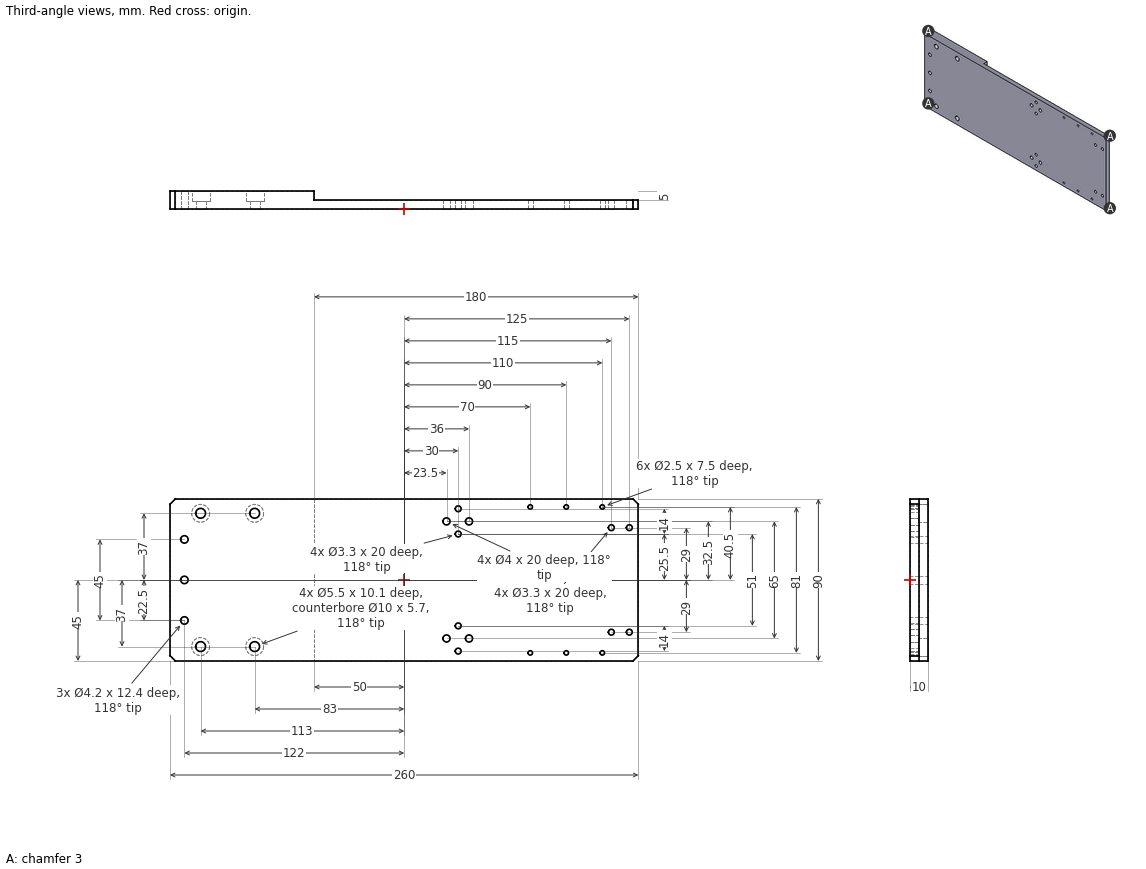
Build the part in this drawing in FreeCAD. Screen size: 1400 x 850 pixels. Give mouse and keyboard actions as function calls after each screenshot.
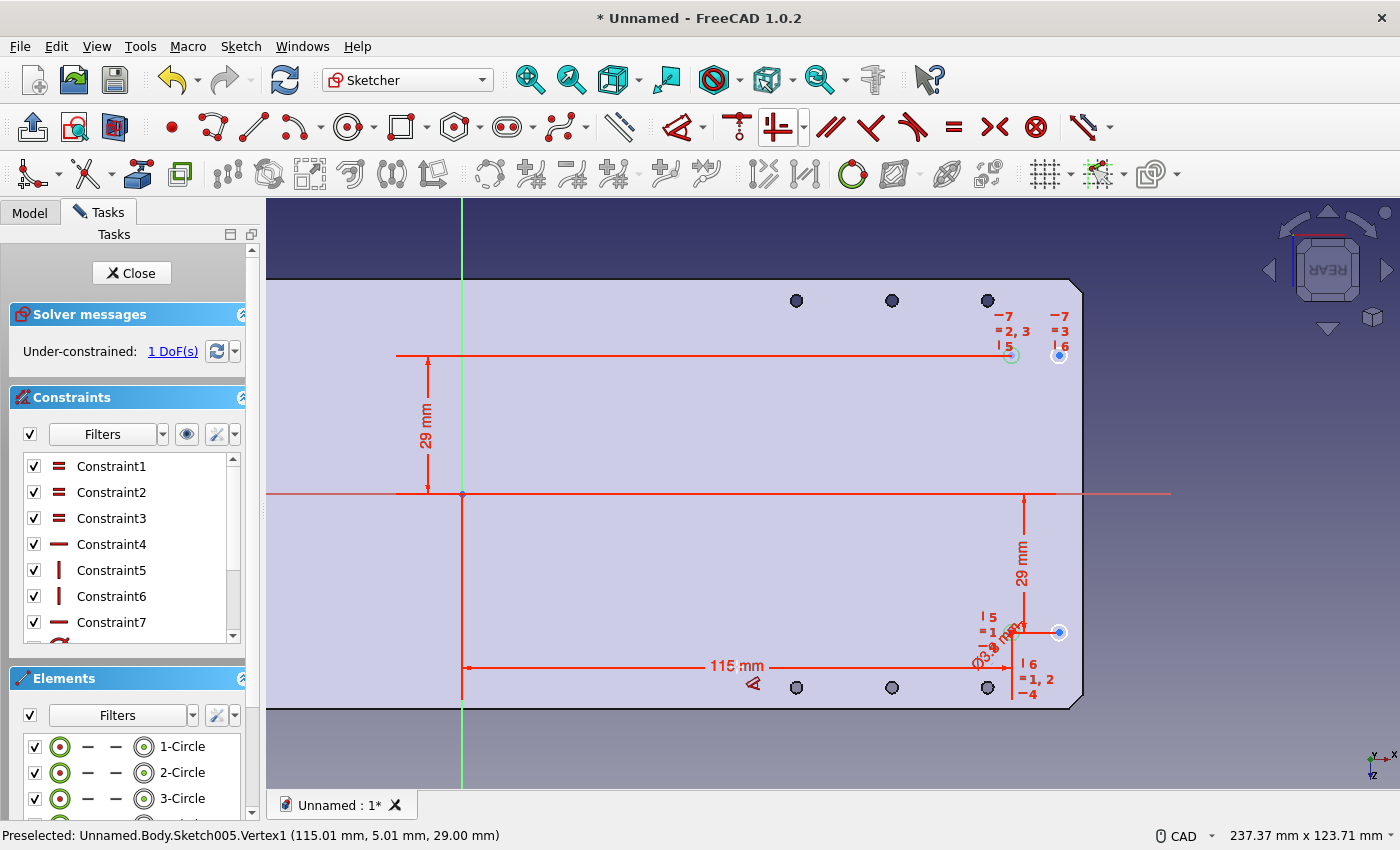
click(1059, 633)
click(623, 667)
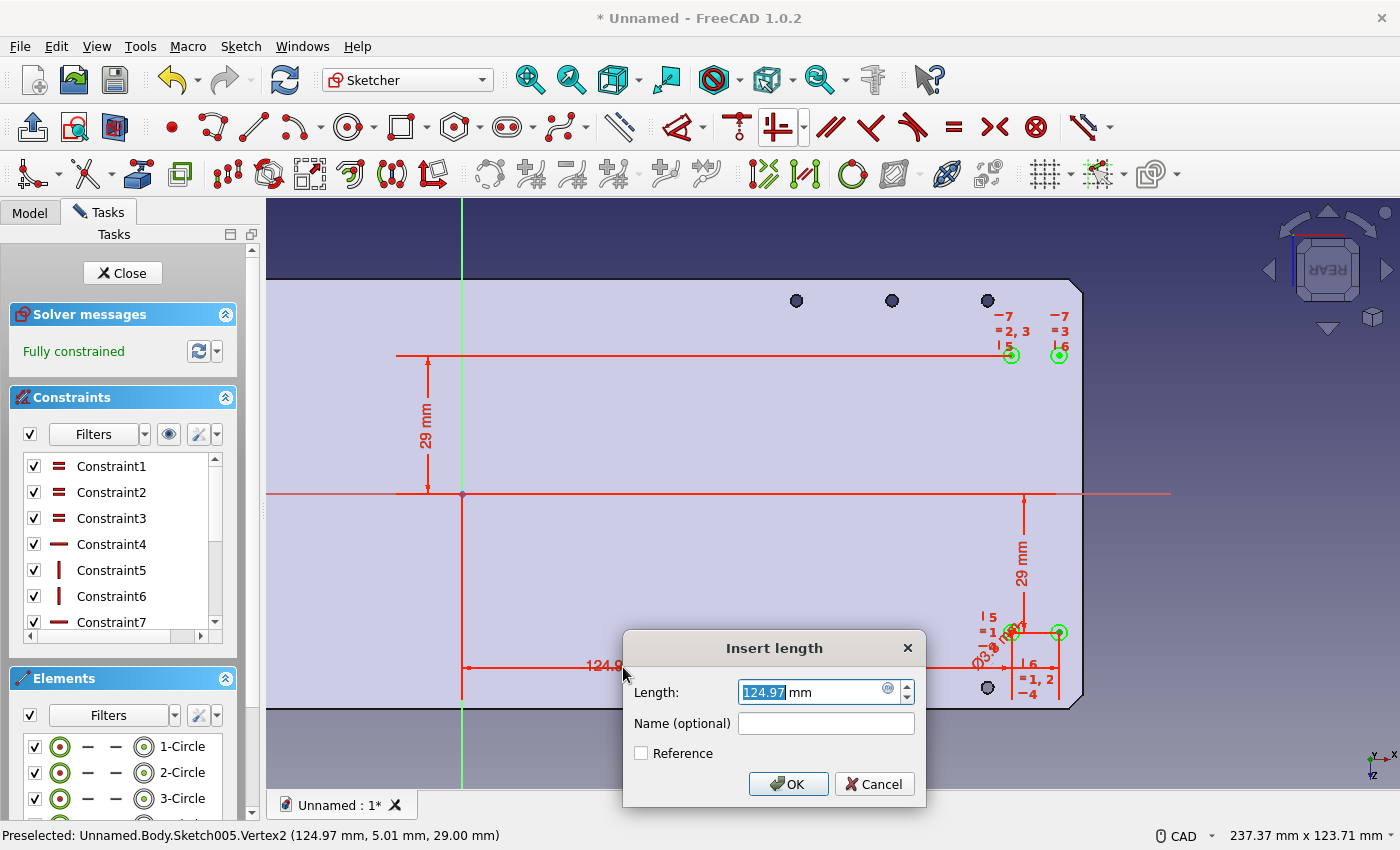
text(125)
key(Return)
key(Escape)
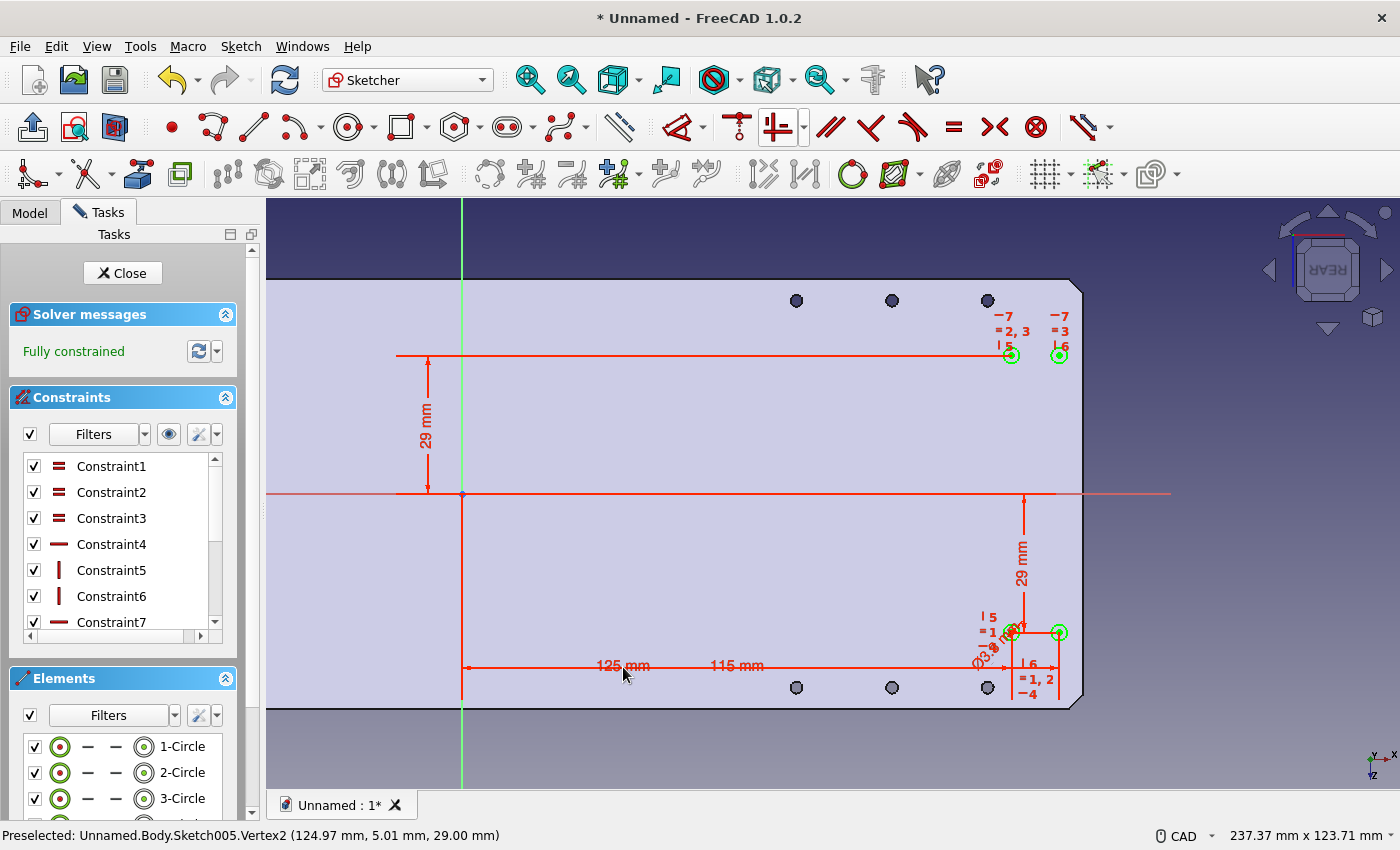
click(123, 273)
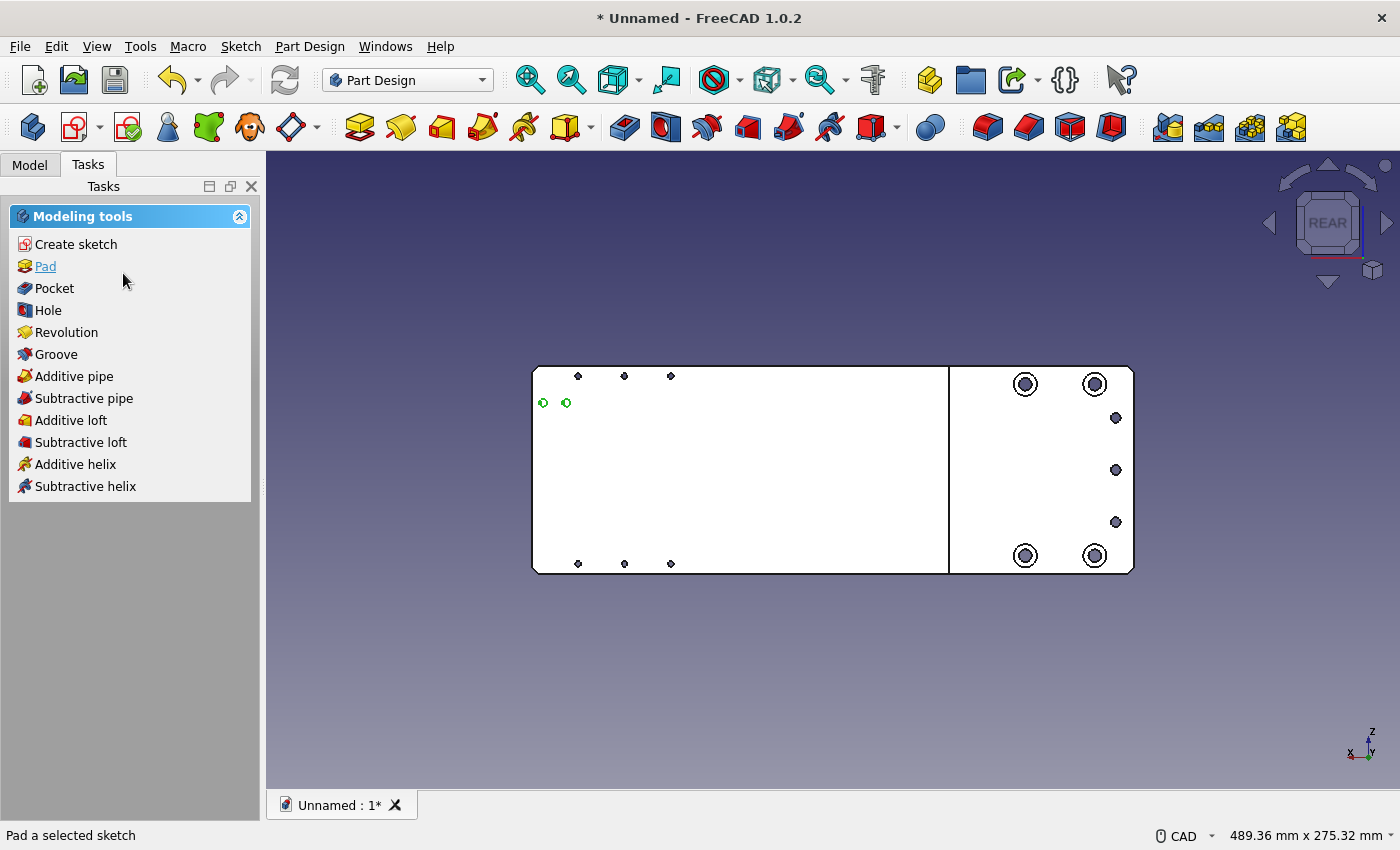
click(666, 128)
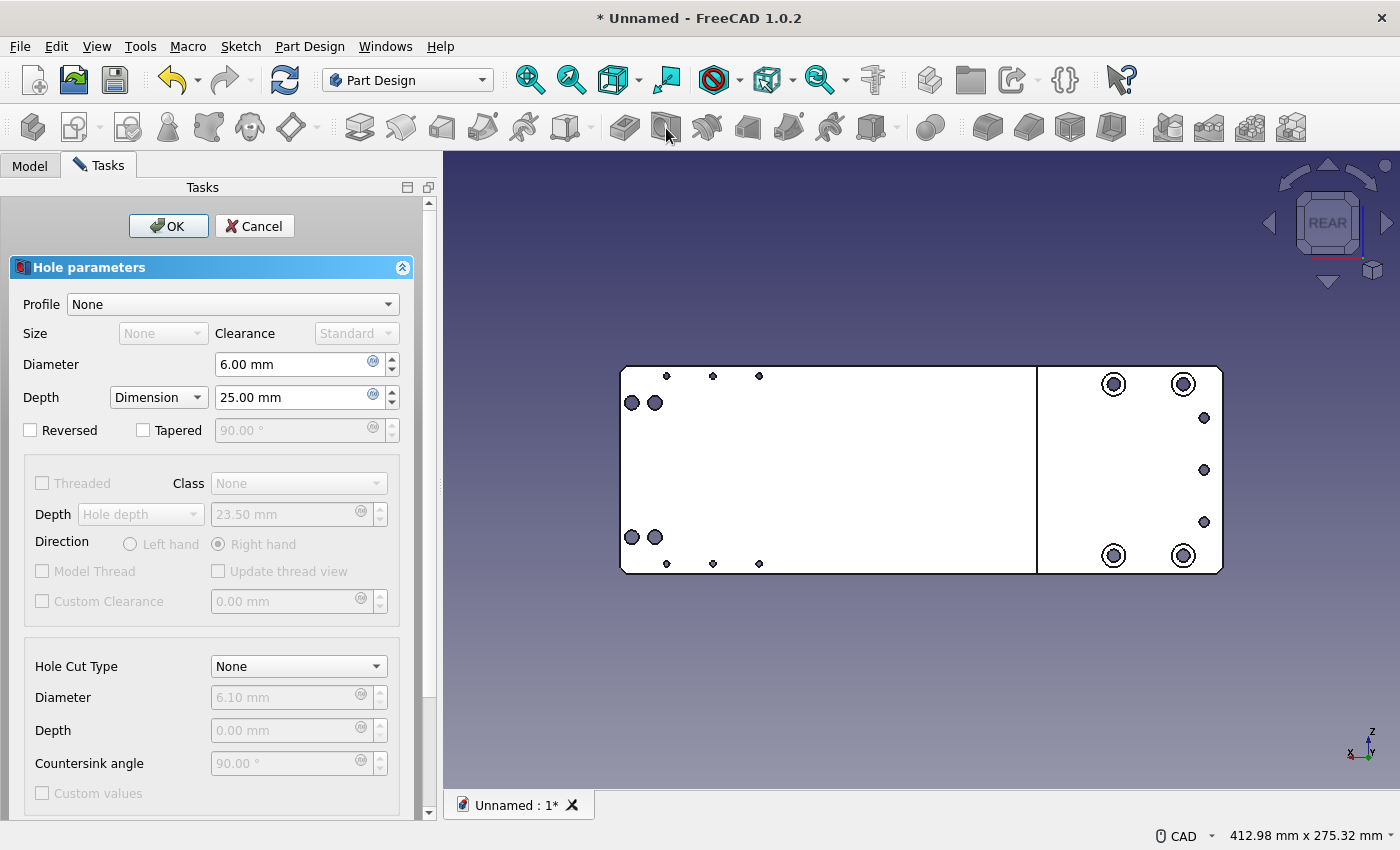
triple_click(300, 364)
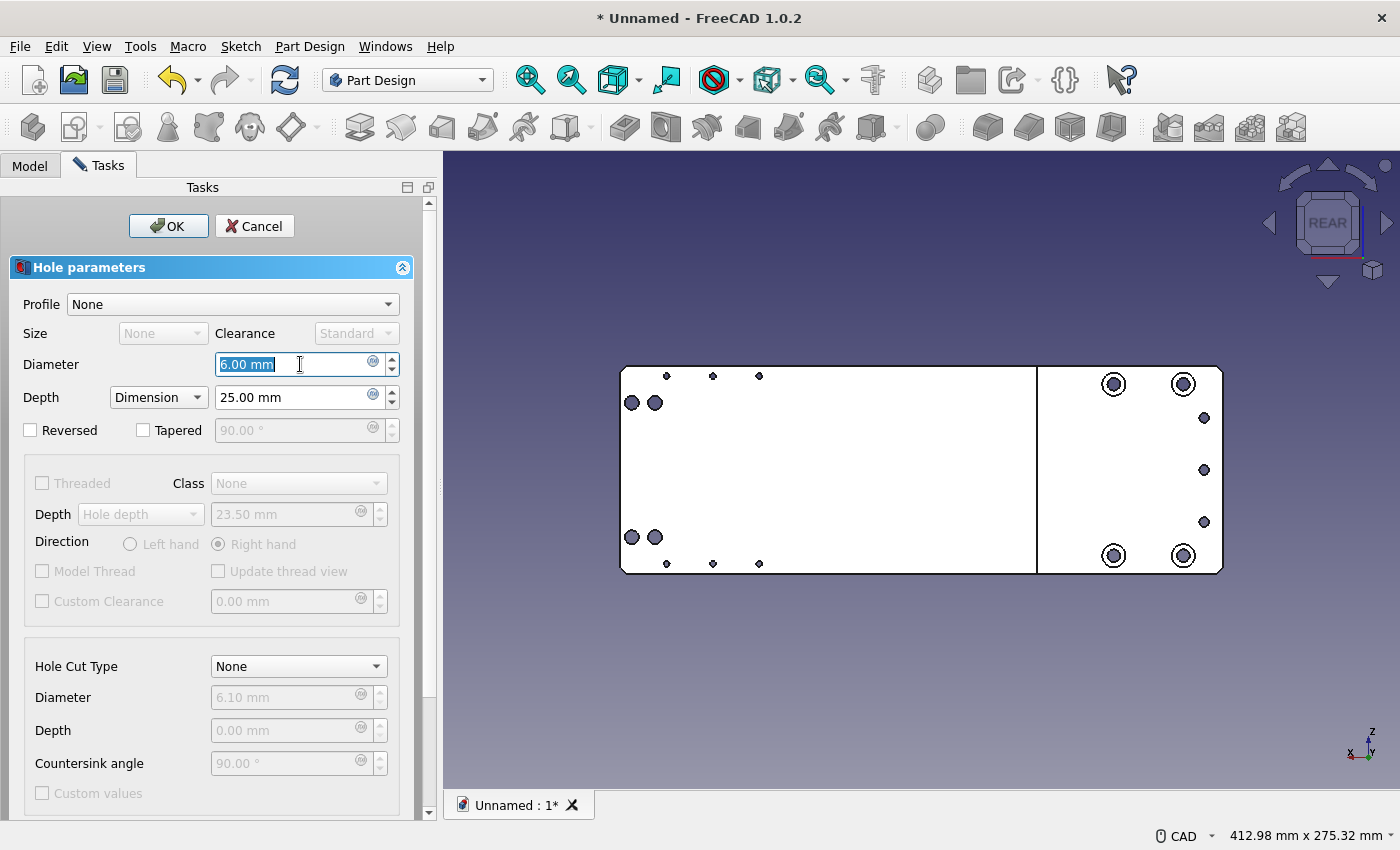
text(3.3)
key(Tab)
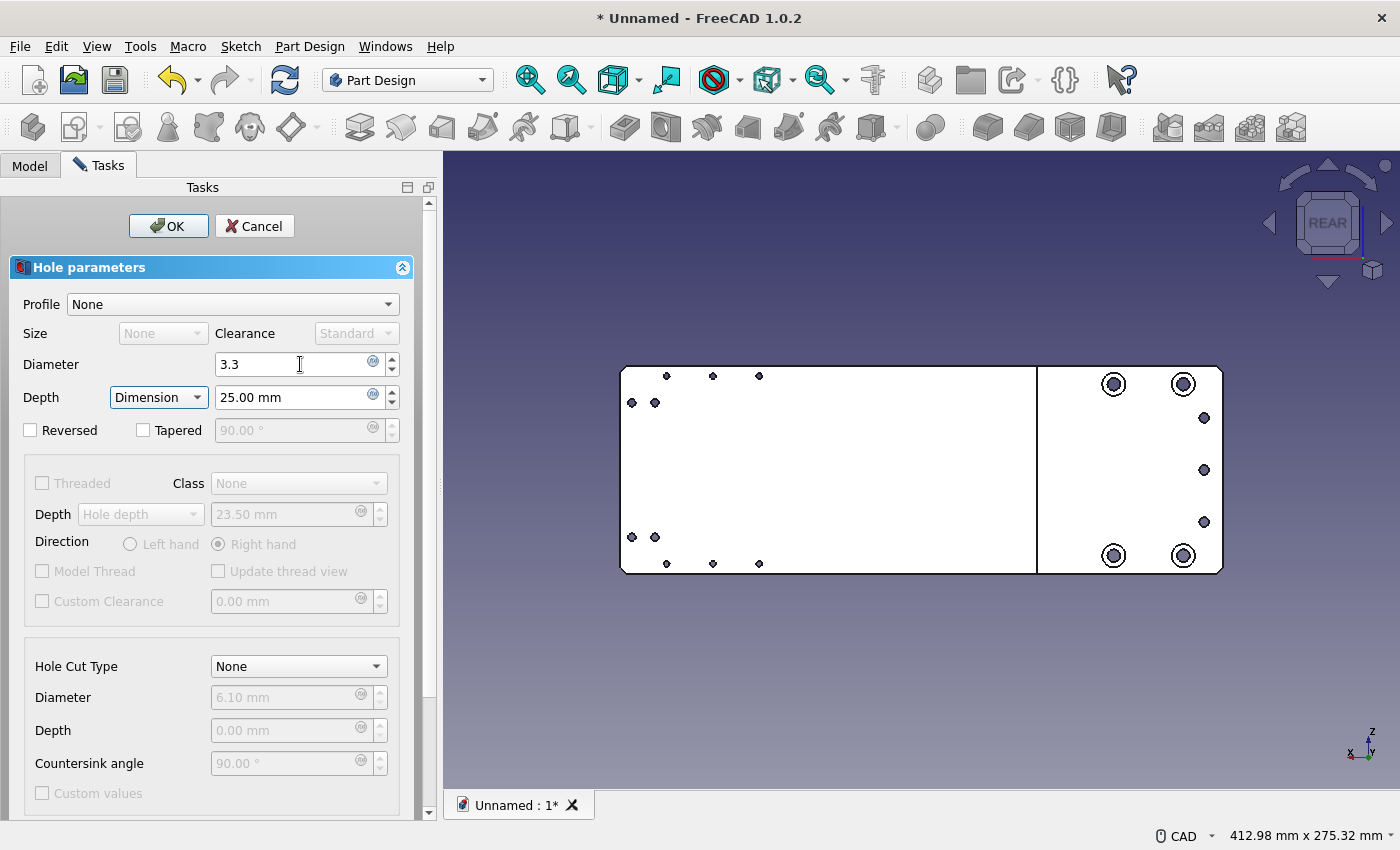
triple_click(300, 398)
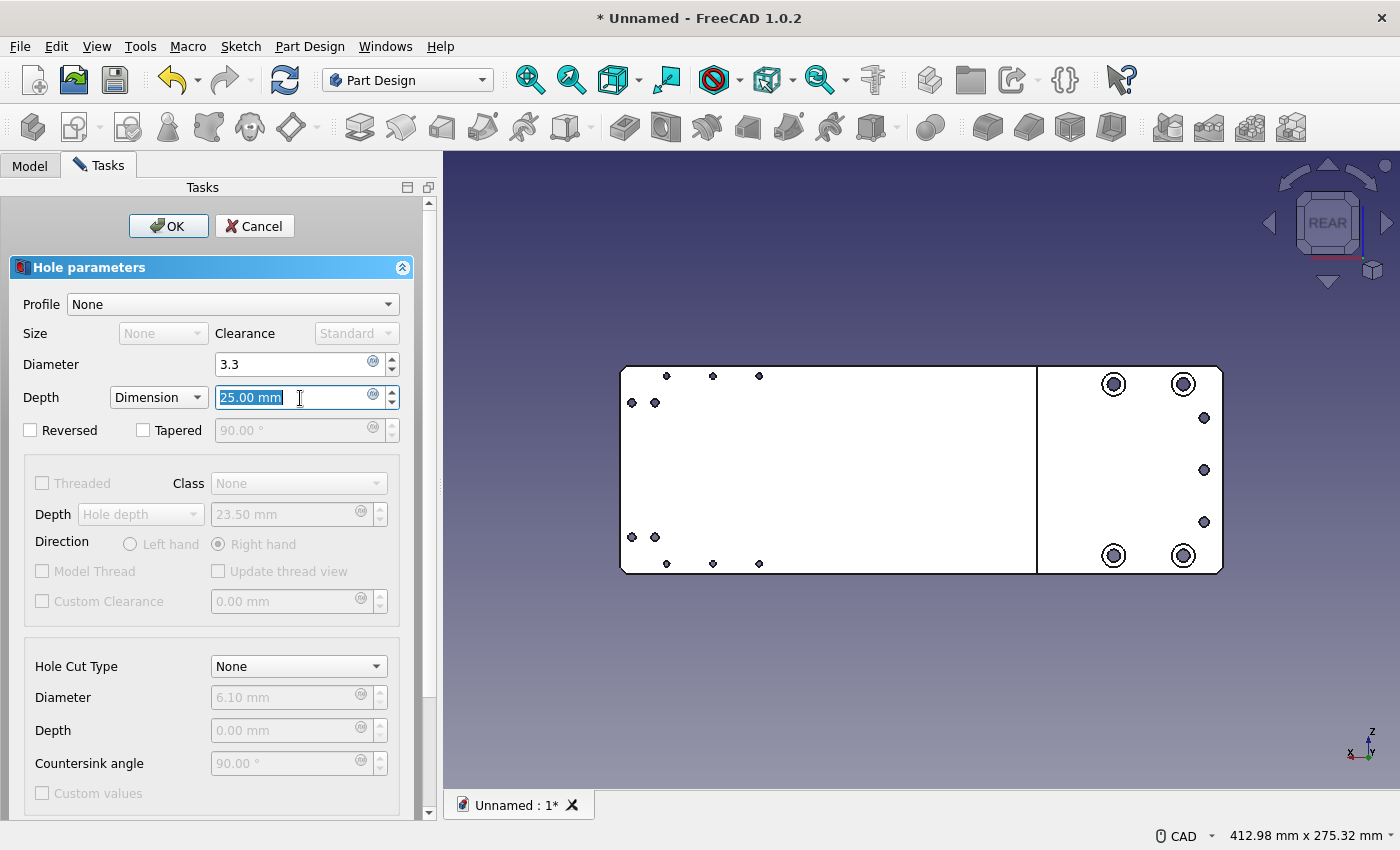
text(20)
key(Tab)